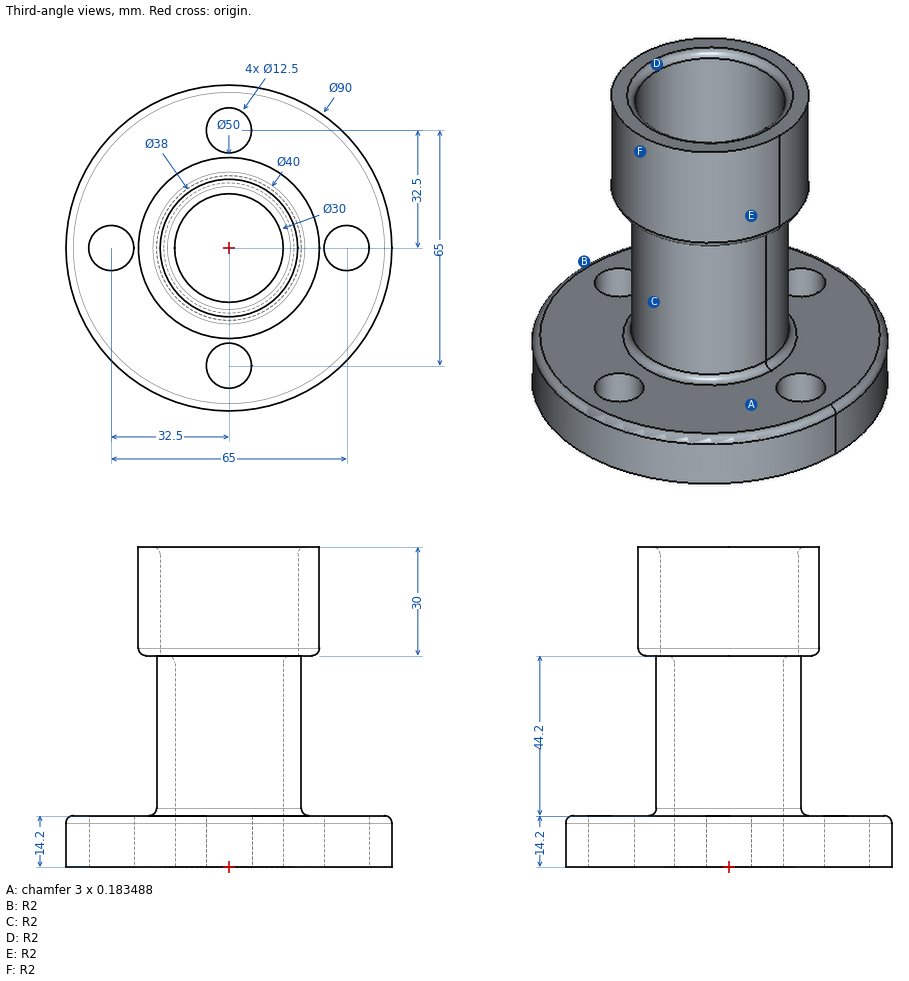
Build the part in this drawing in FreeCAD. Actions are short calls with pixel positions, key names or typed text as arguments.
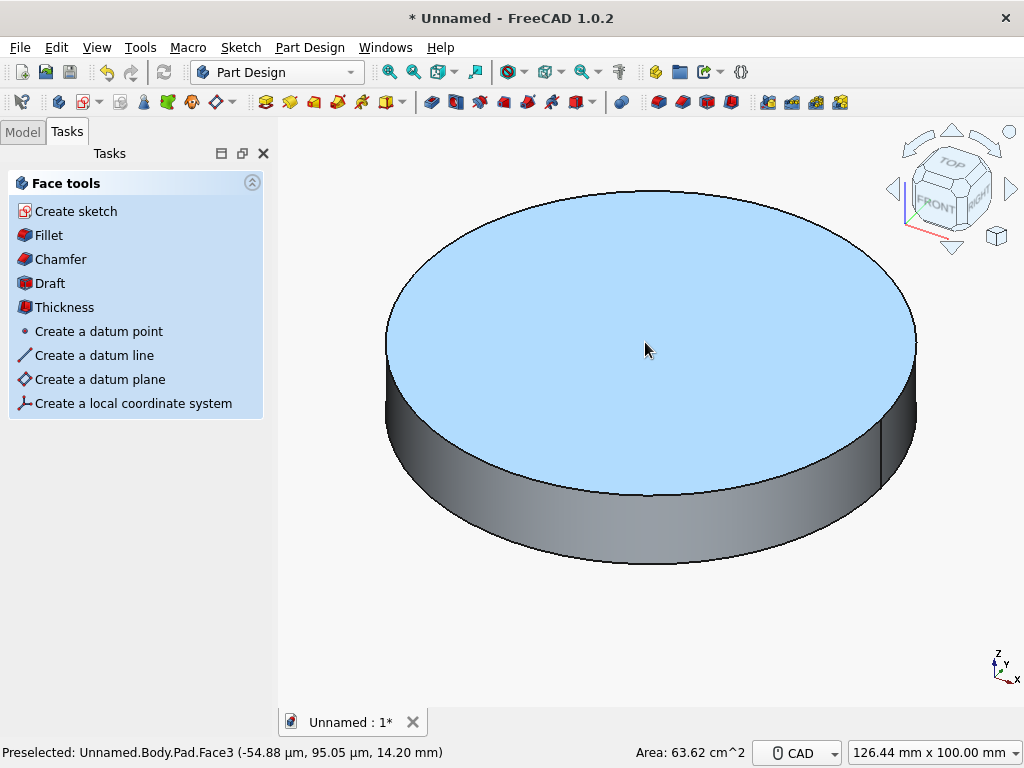
click(84, 102)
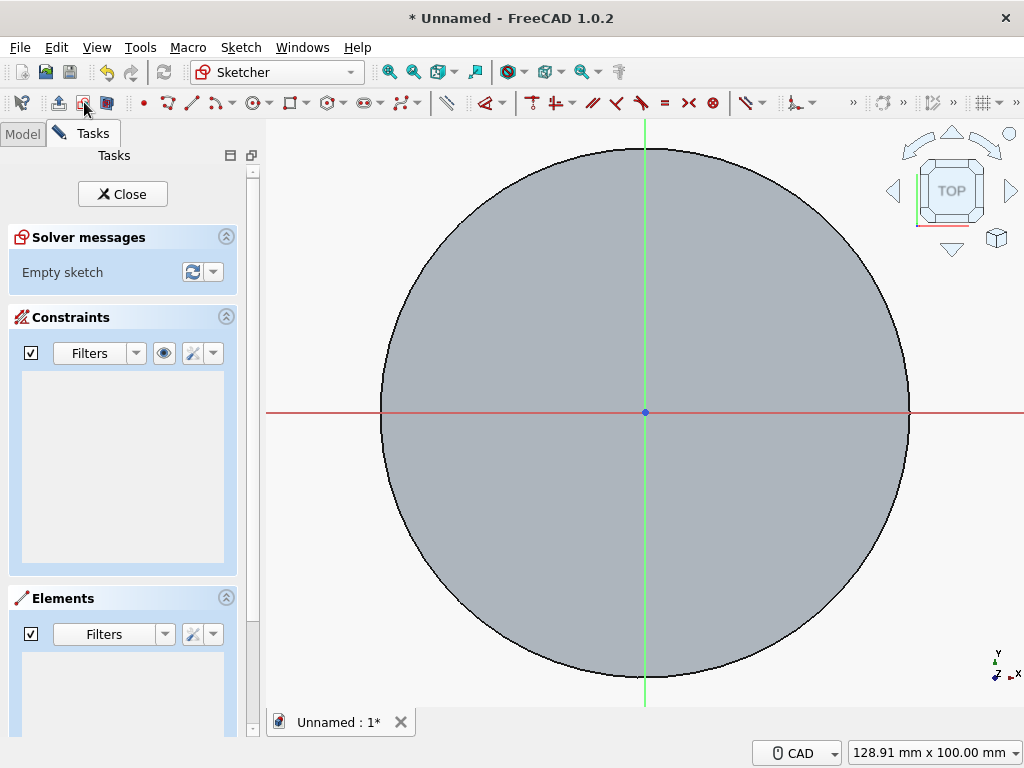
scroll(294, 413, down, 1)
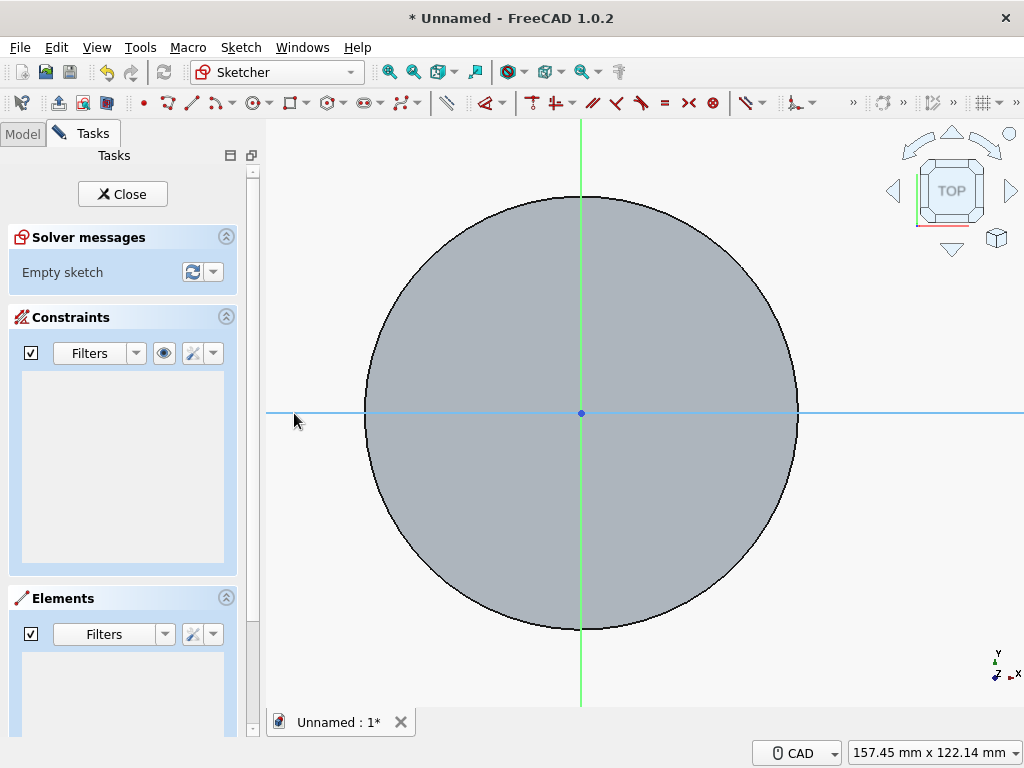
click(254, 104)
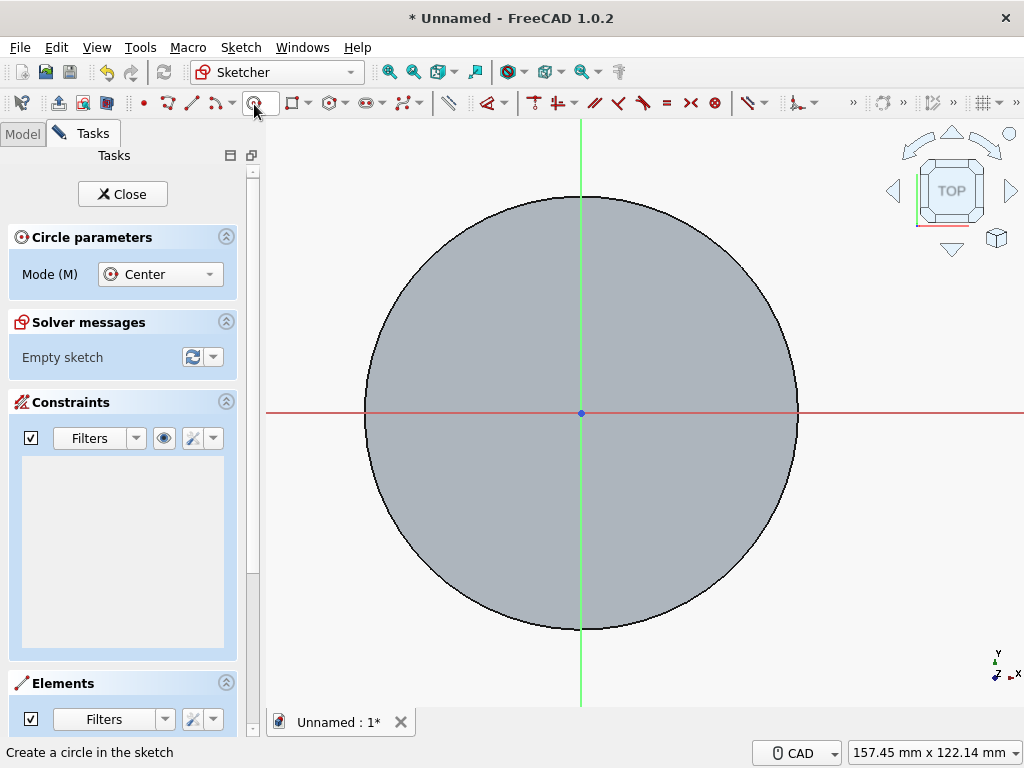
click(581, 257)
move(603, 235)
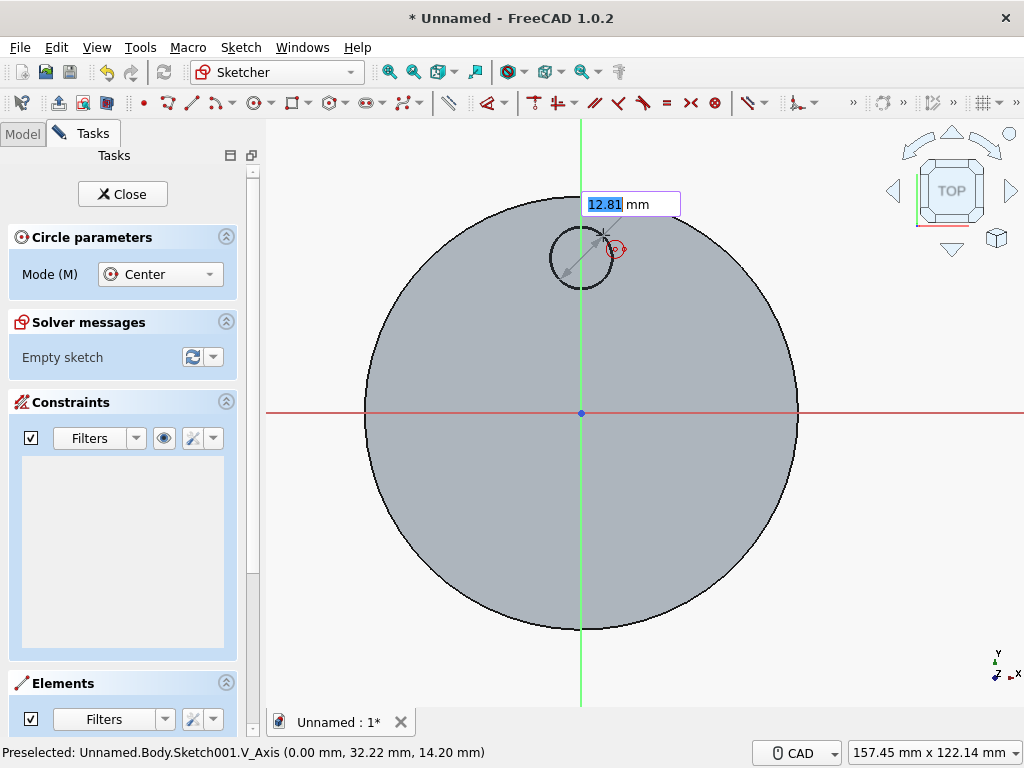
text(12.5)
key(Return)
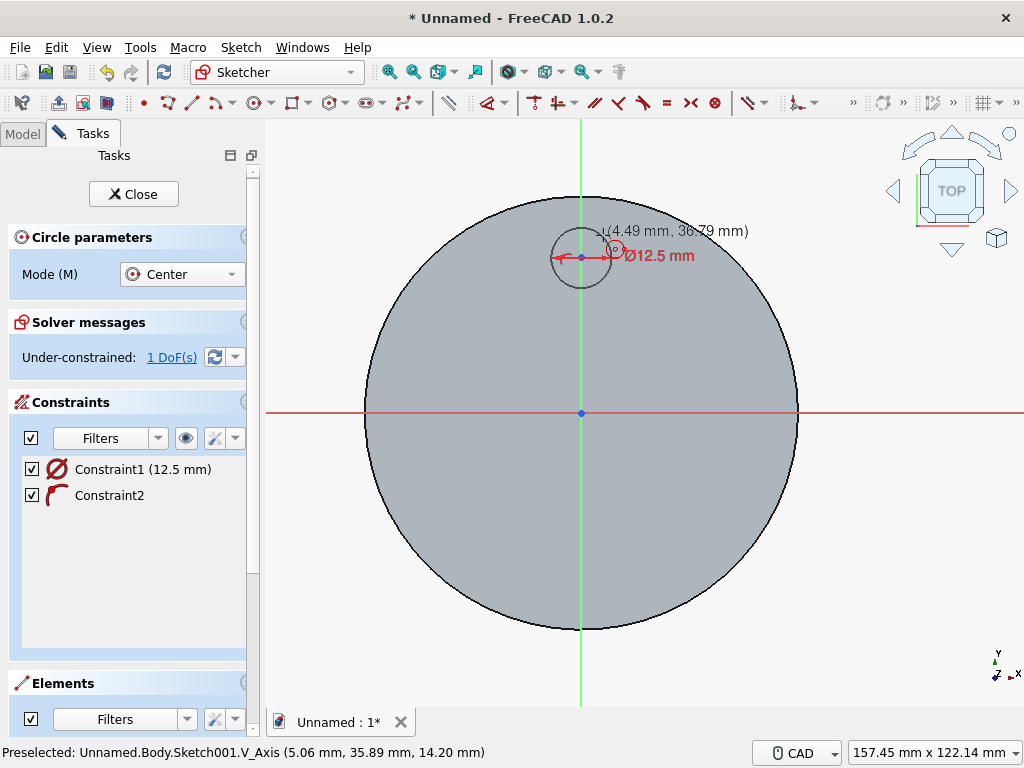
click(581, 570)
move(603, 548)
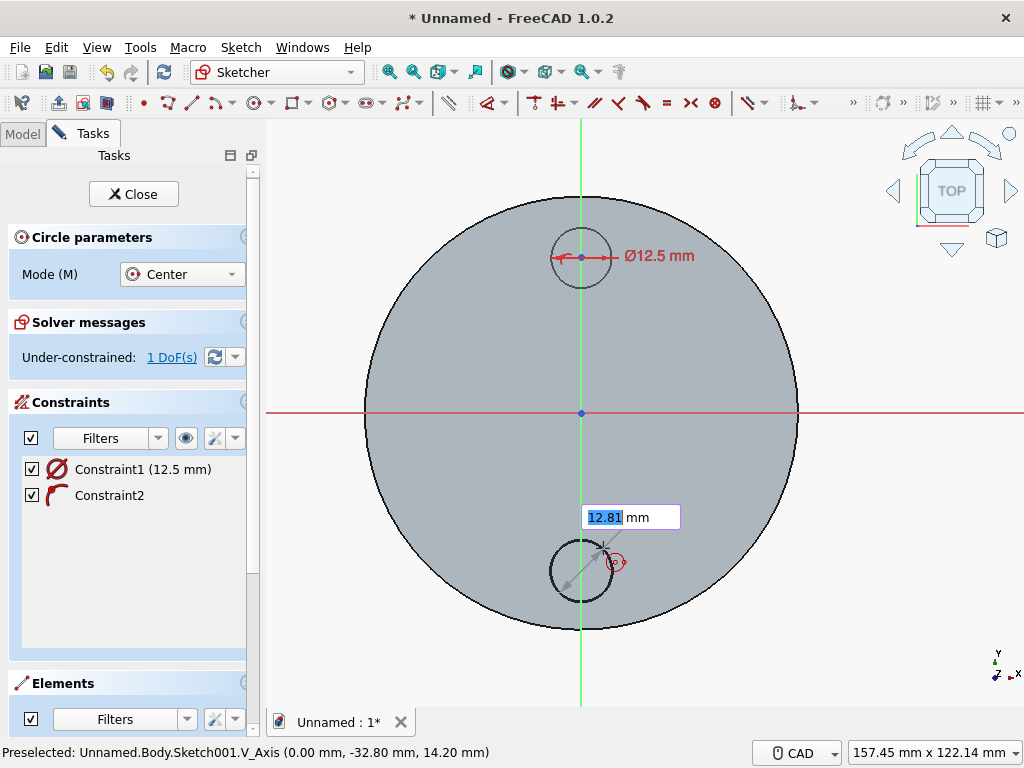
text(12.5)
key(Return)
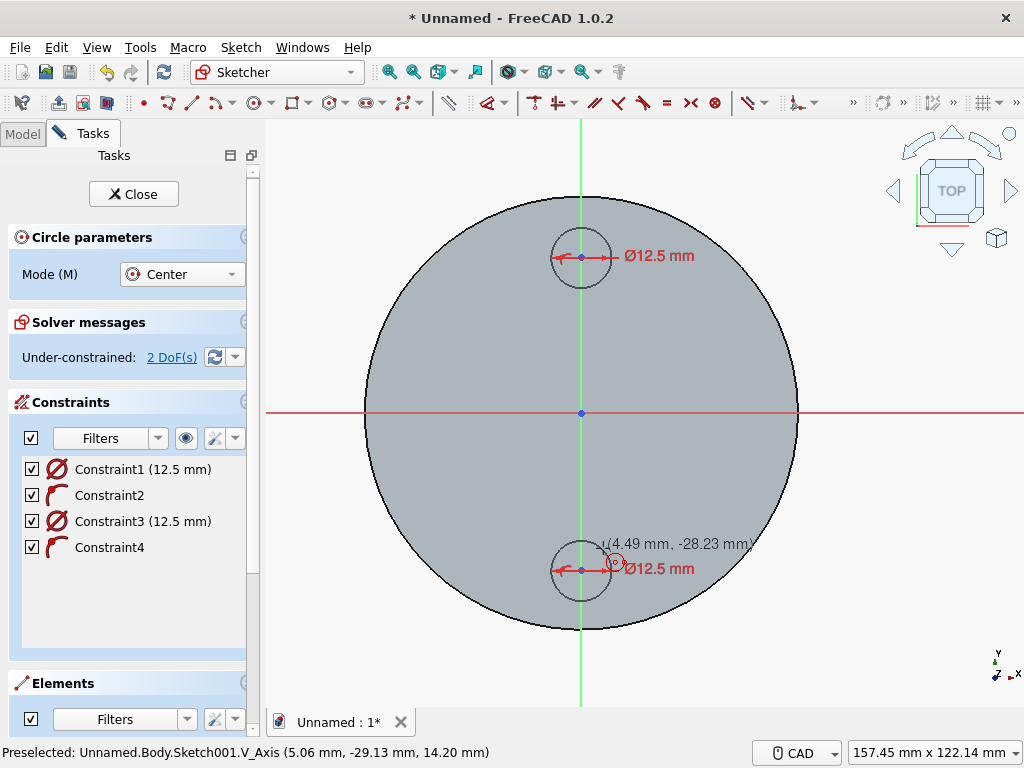
click(425, 413)
move(446, 392)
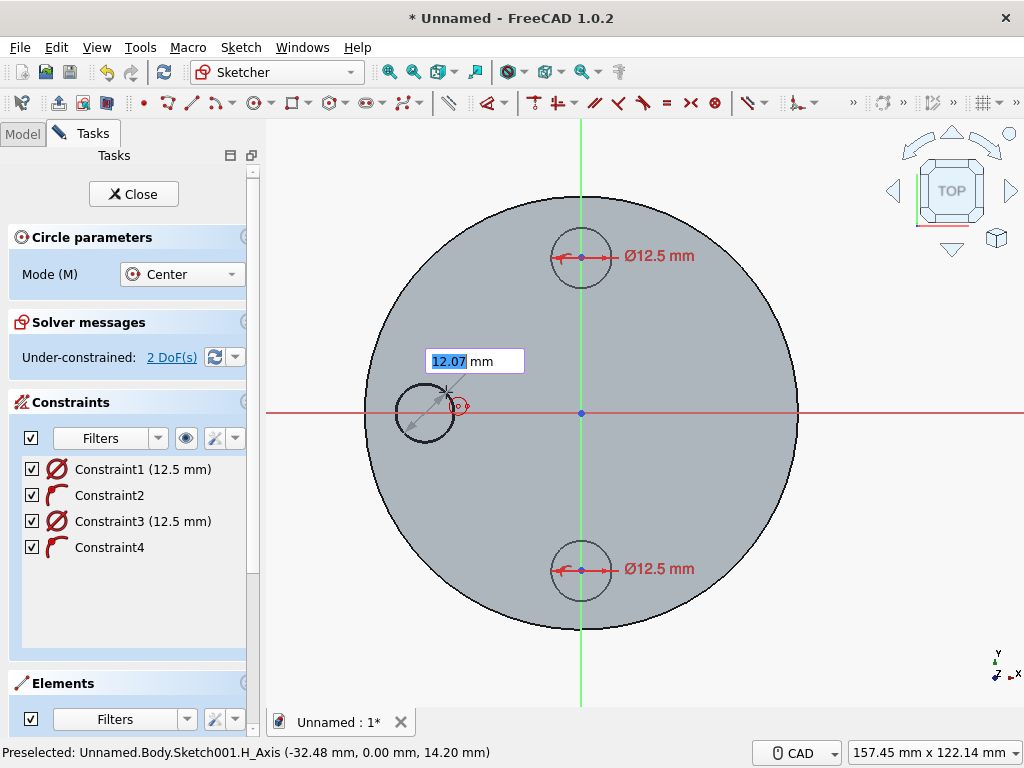
text(12.5)
key(Return)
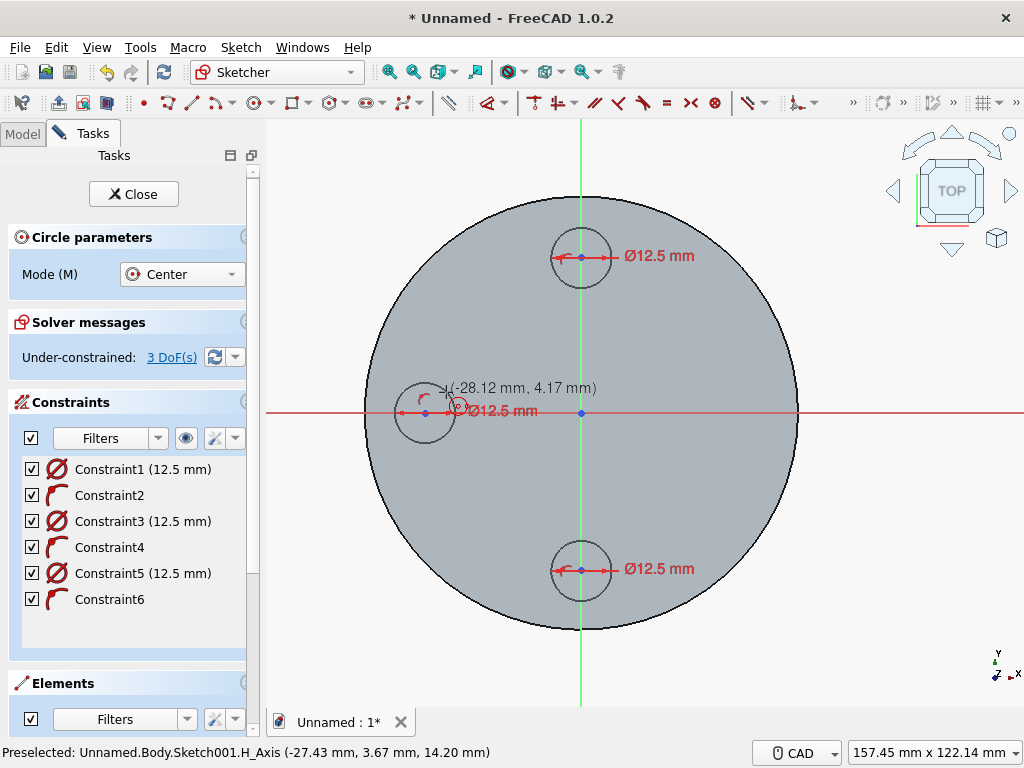
click(738, 413)
move(759, 392)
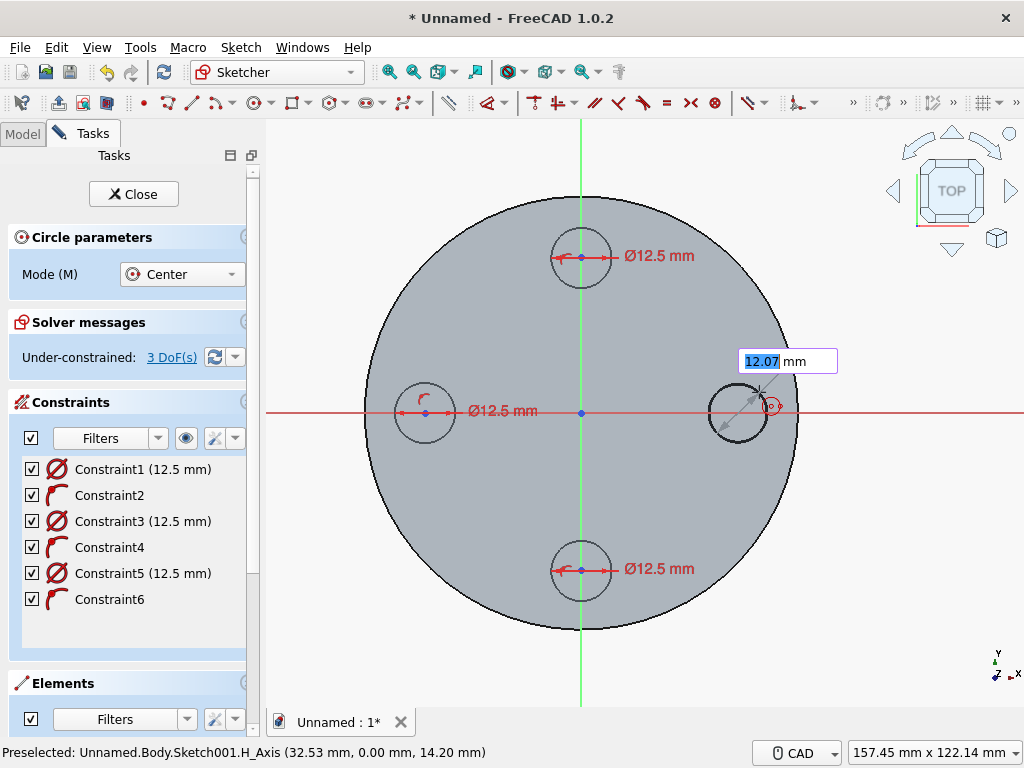
text(12.5)
key(Return)
key(Escape)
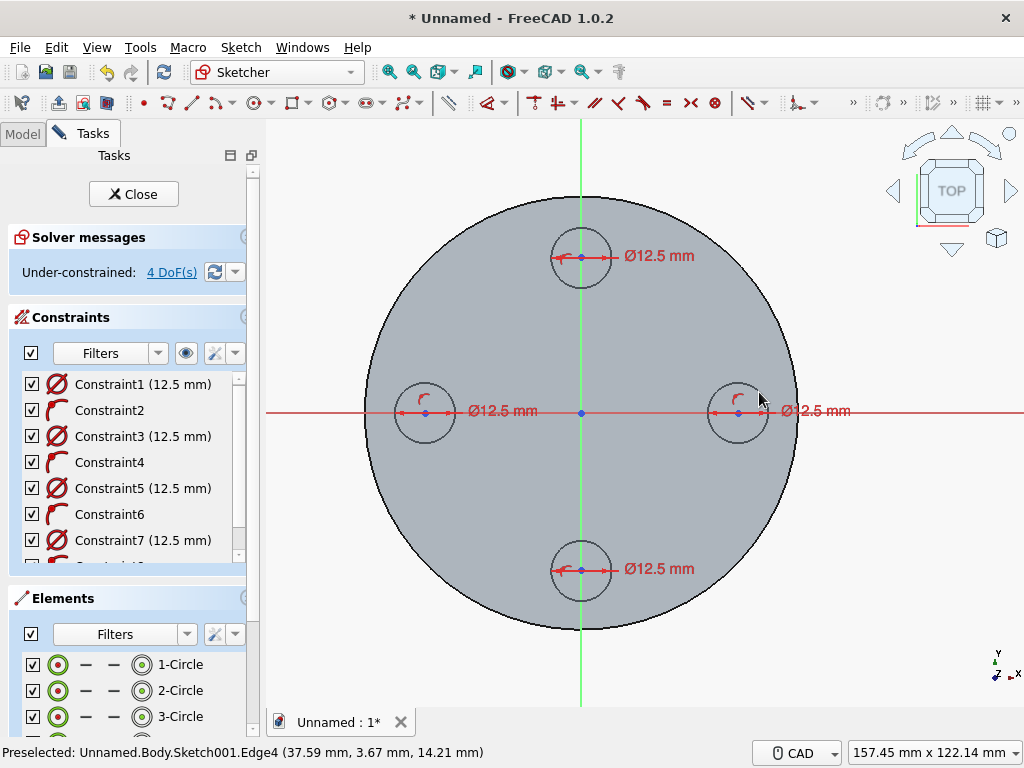
key(d)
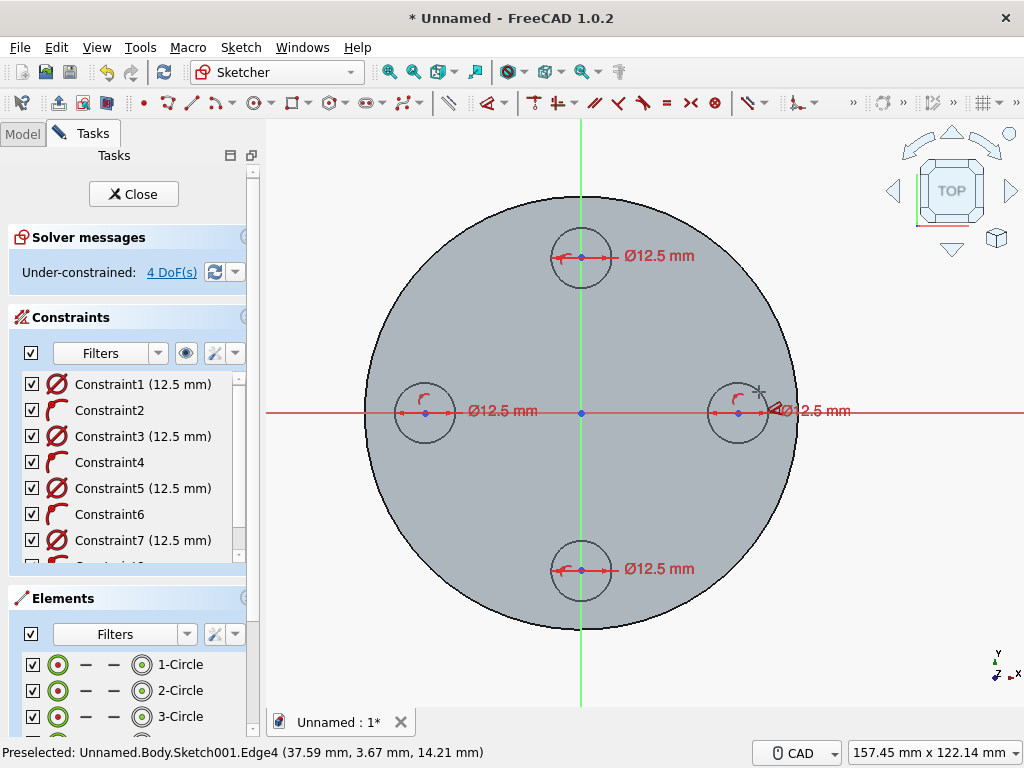
click(581, 258)